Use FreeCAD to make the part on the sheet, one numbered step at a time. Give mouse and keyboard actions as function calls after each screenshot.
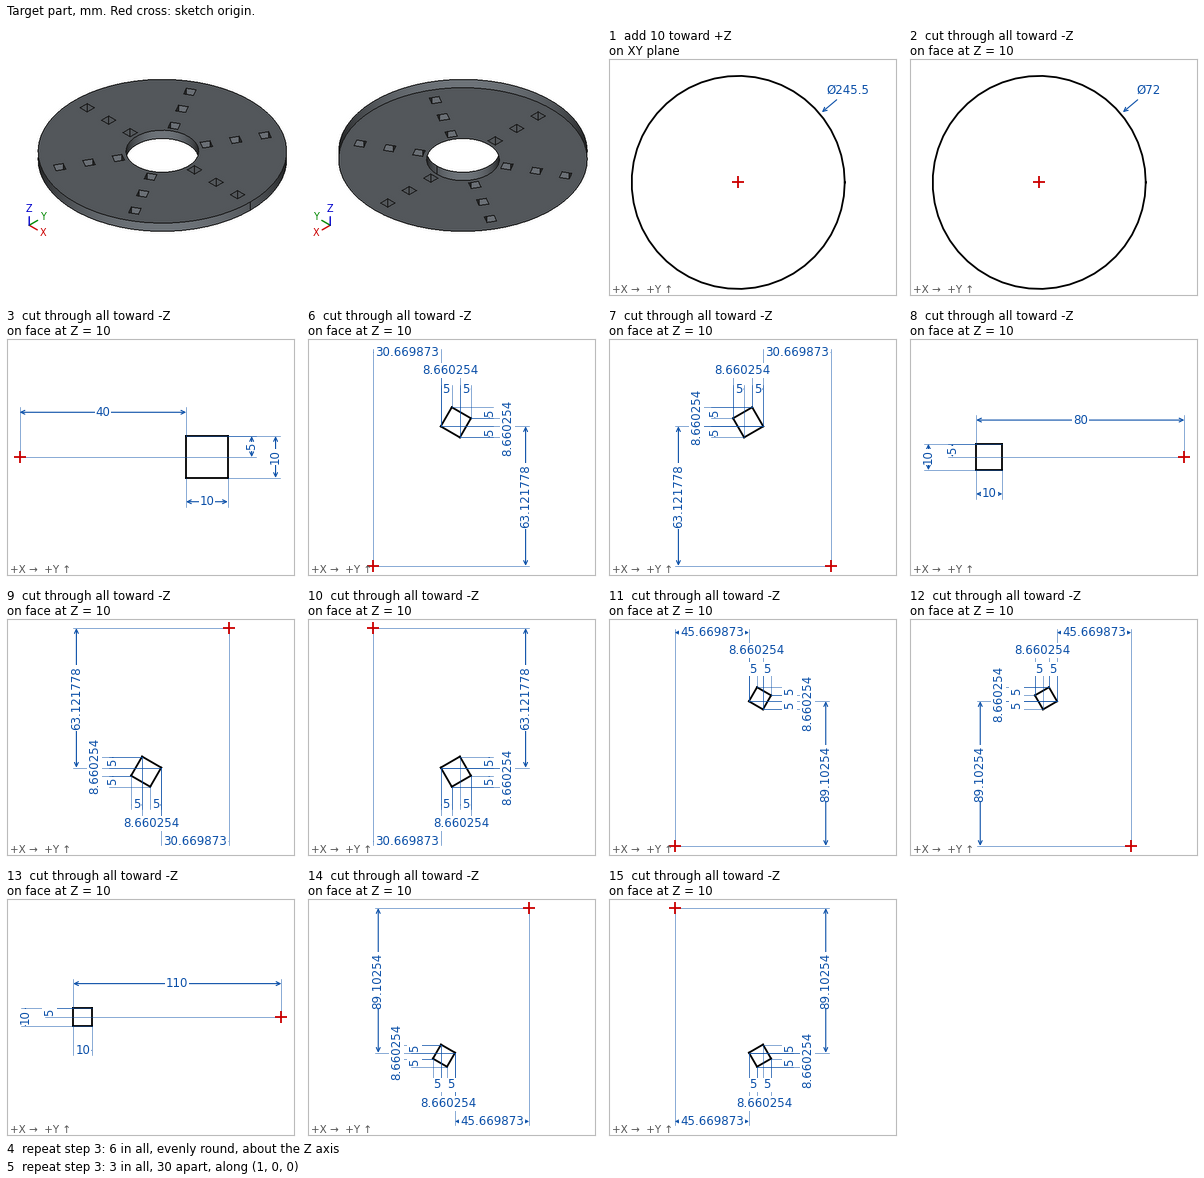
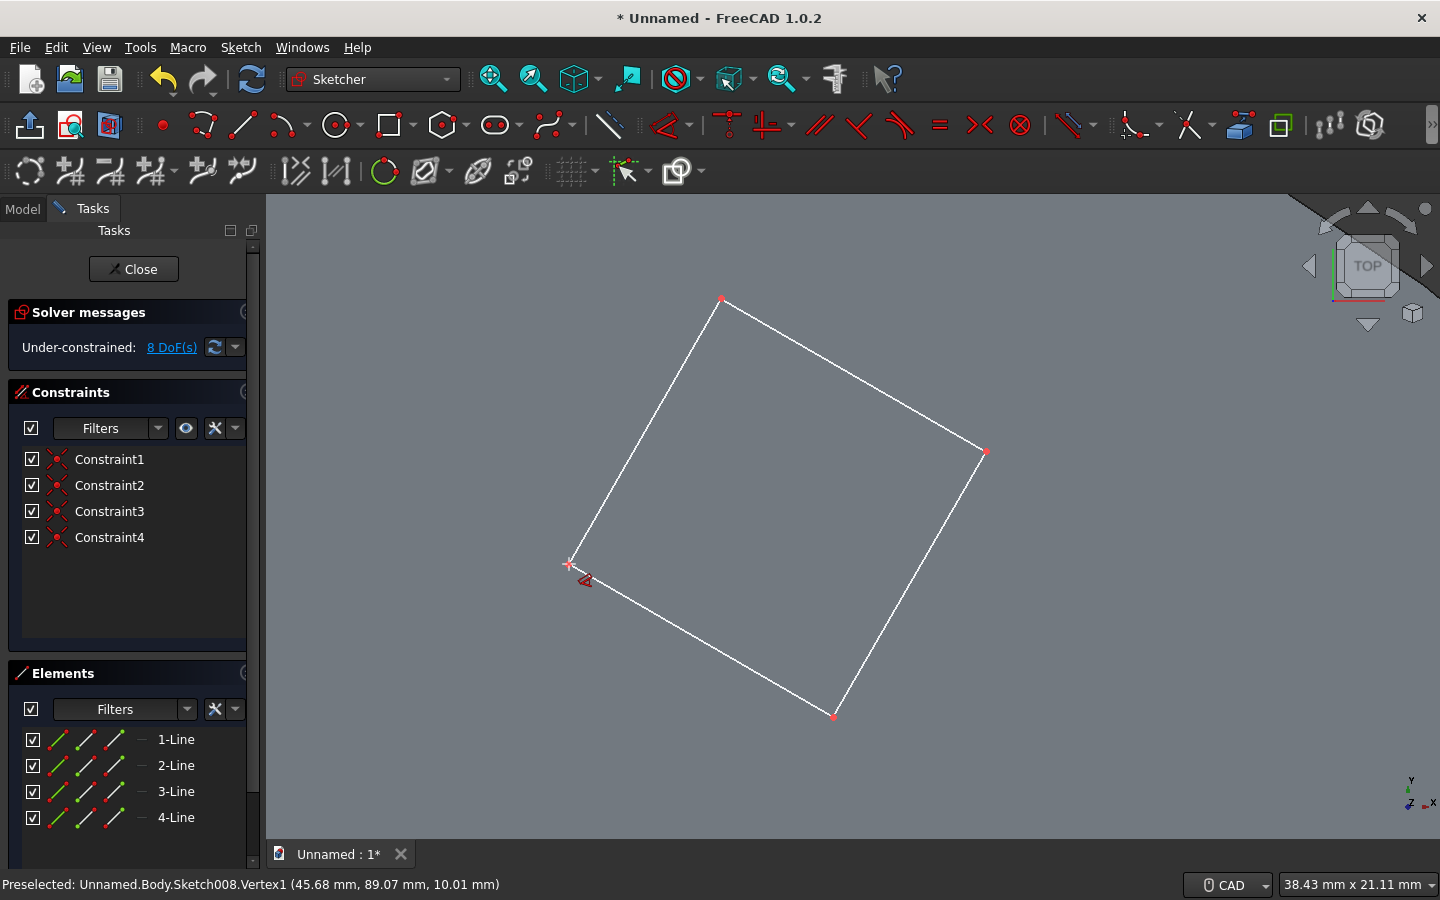
click(648, 610)
click(535, 641)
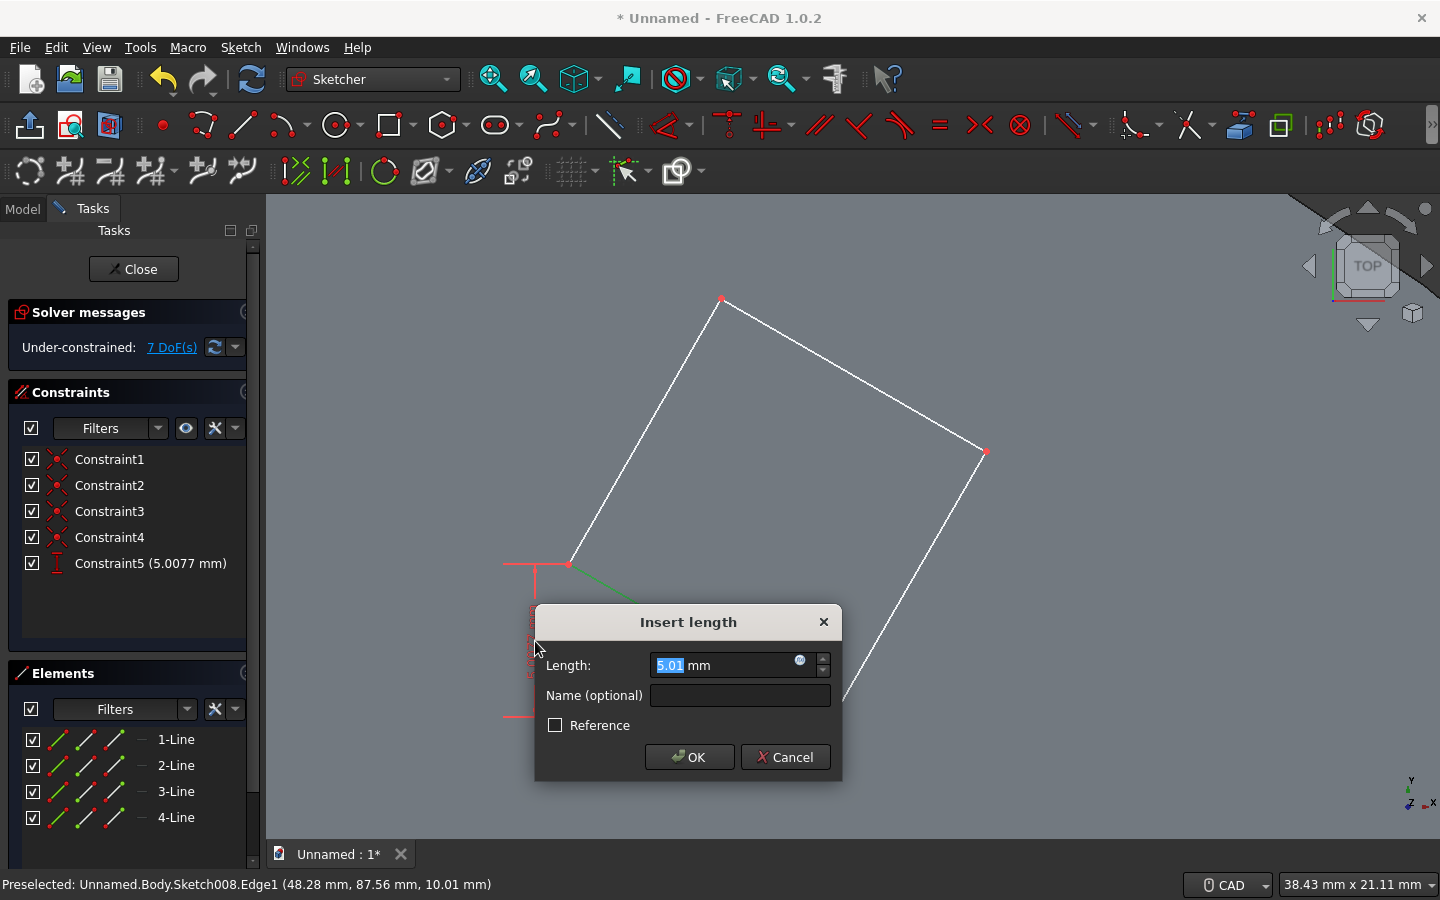
text(5)
key(Return)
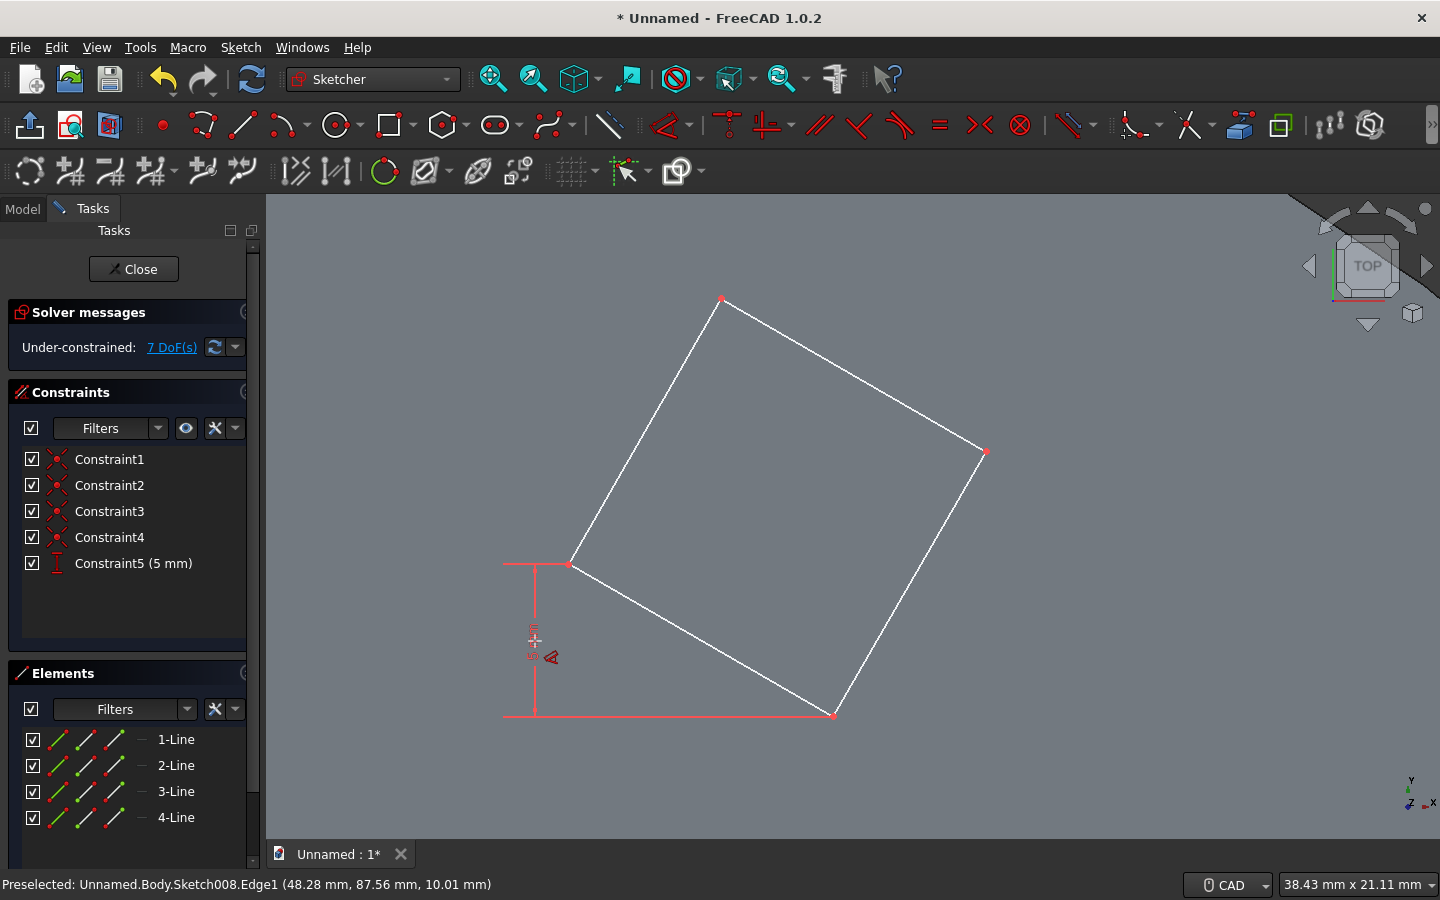
click(879, 637)
click(909, 751)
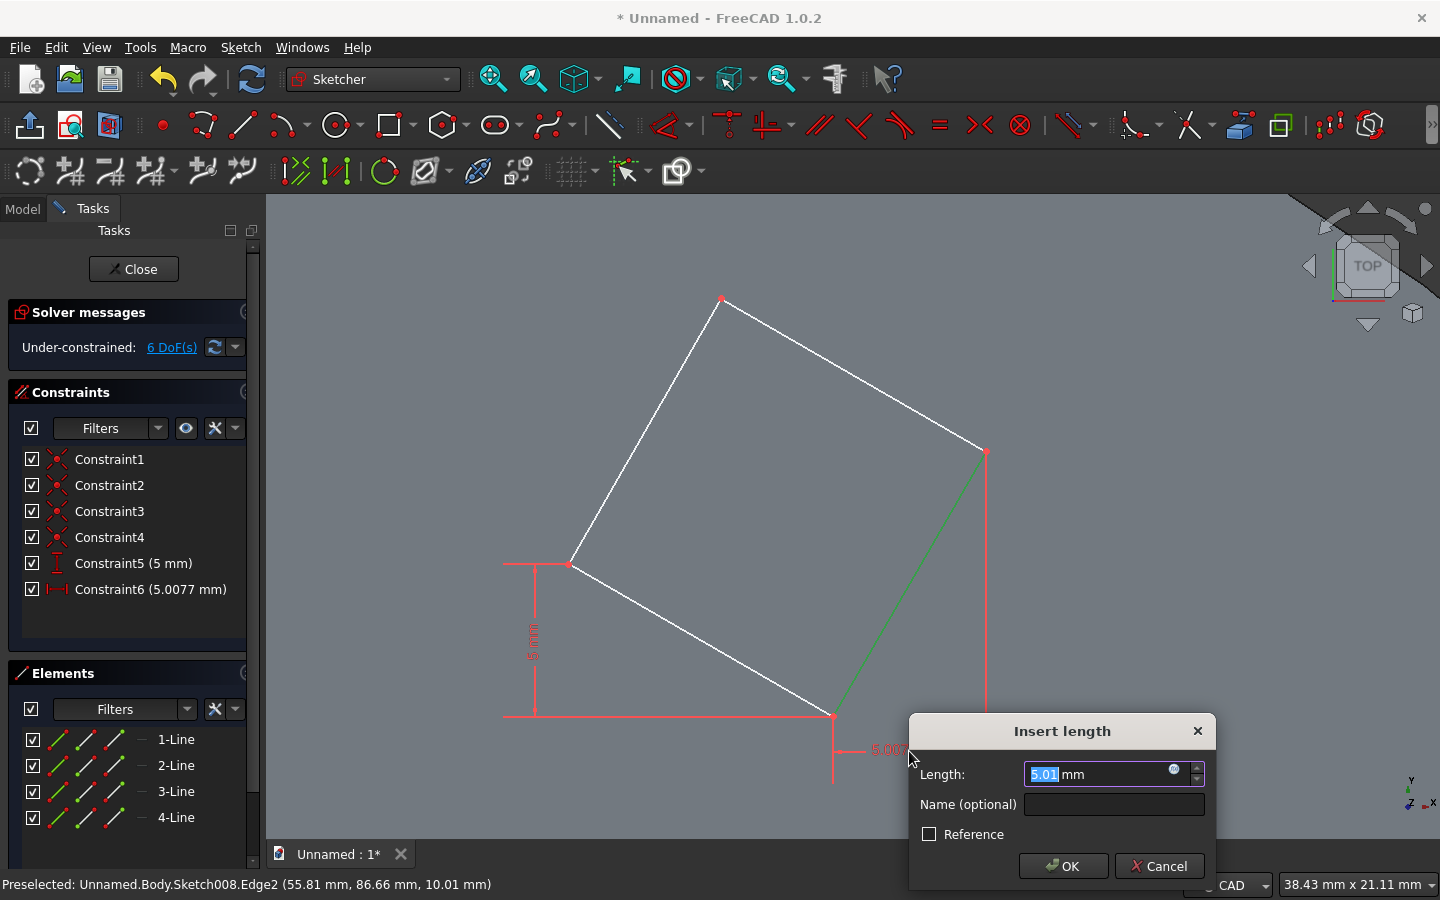
text(5)
key(Return)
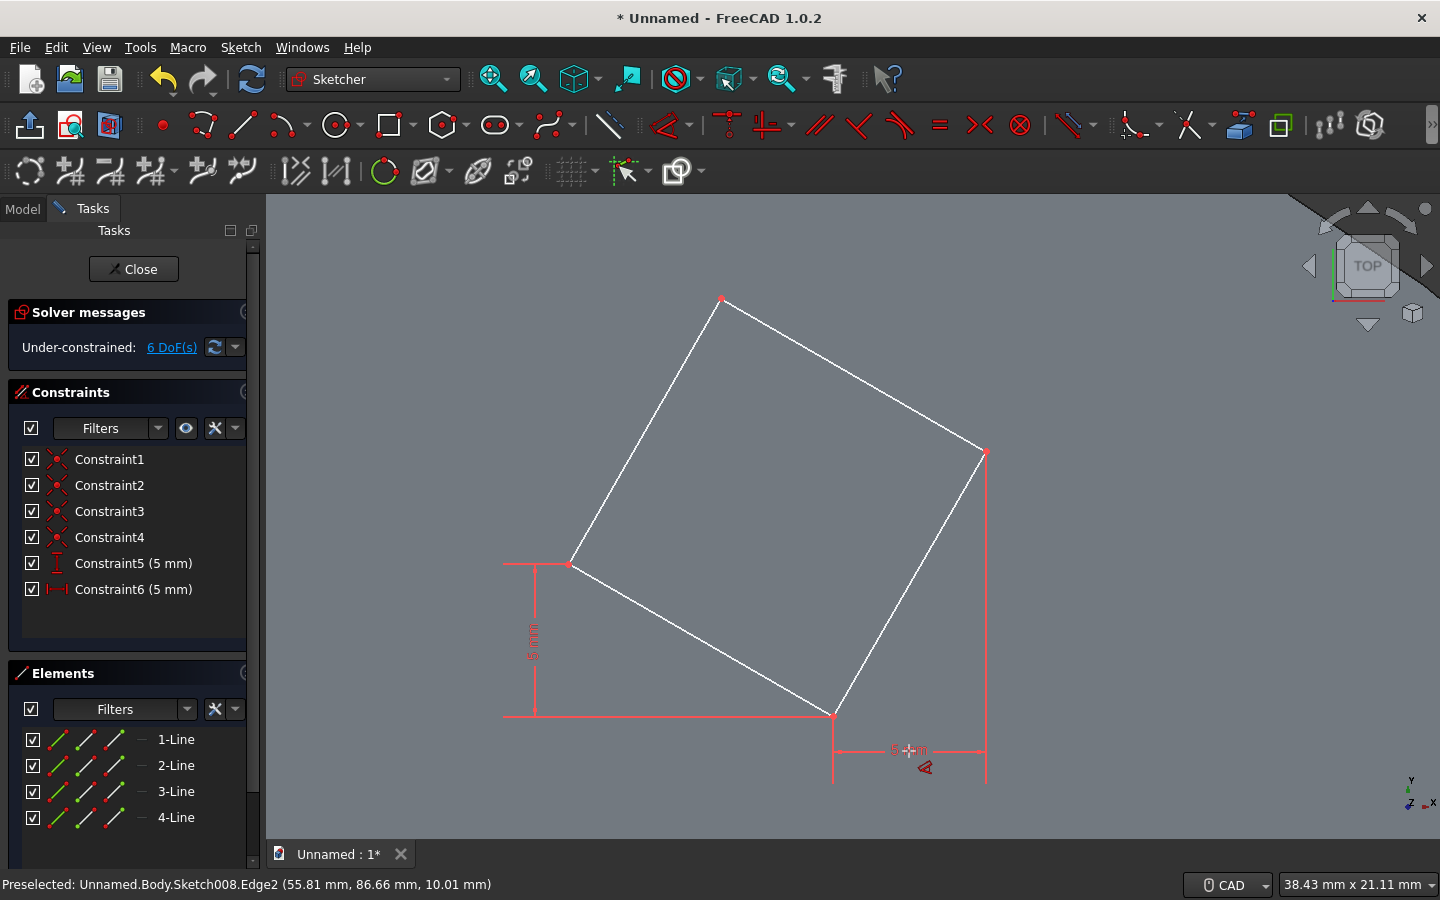
click(907, 406)
click(1020, 375)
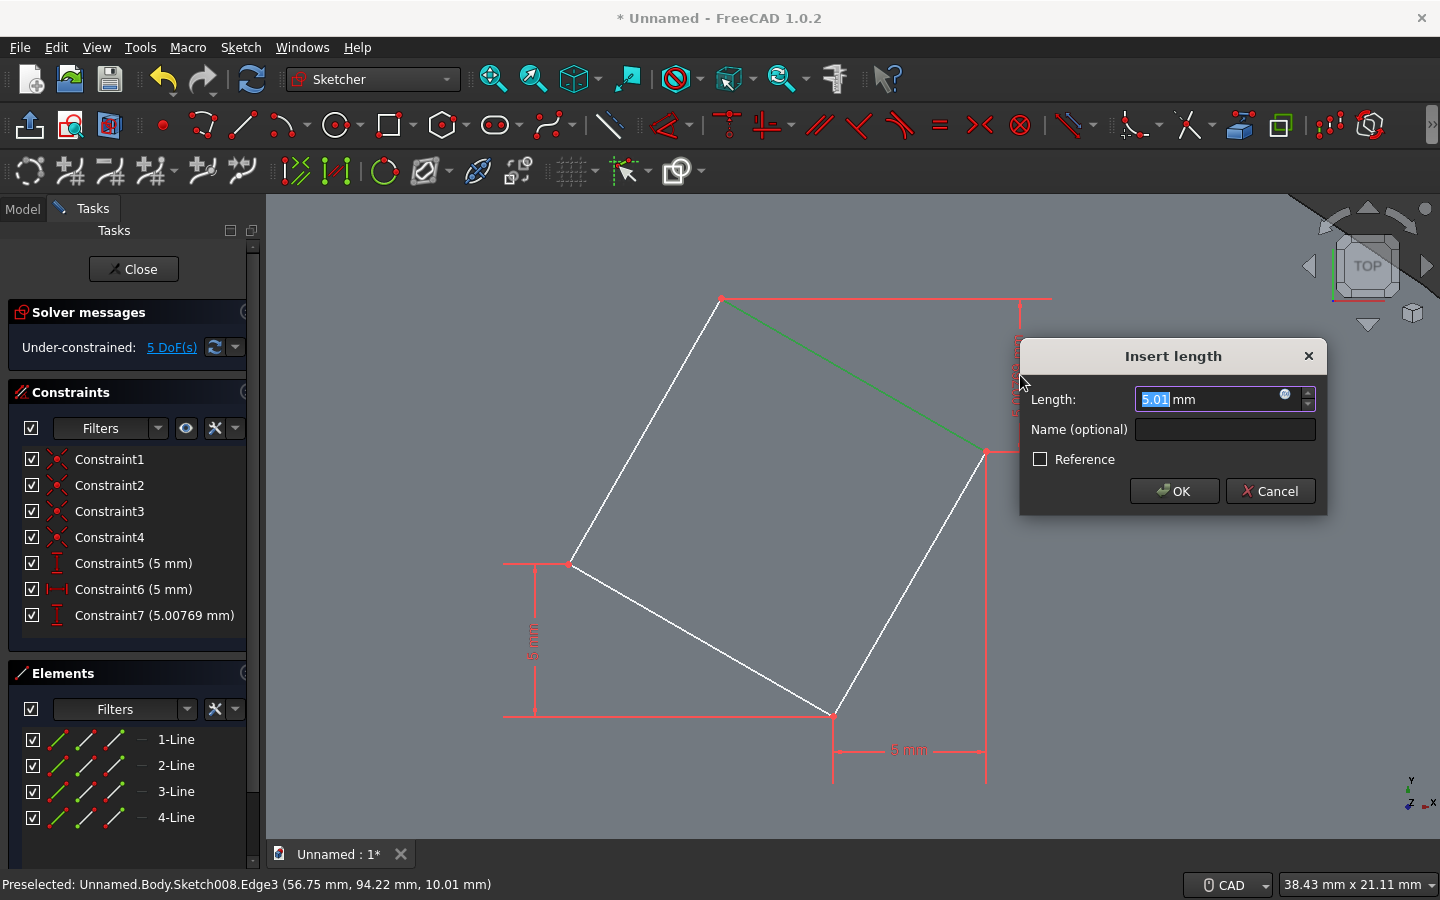
text(5)
key(Return)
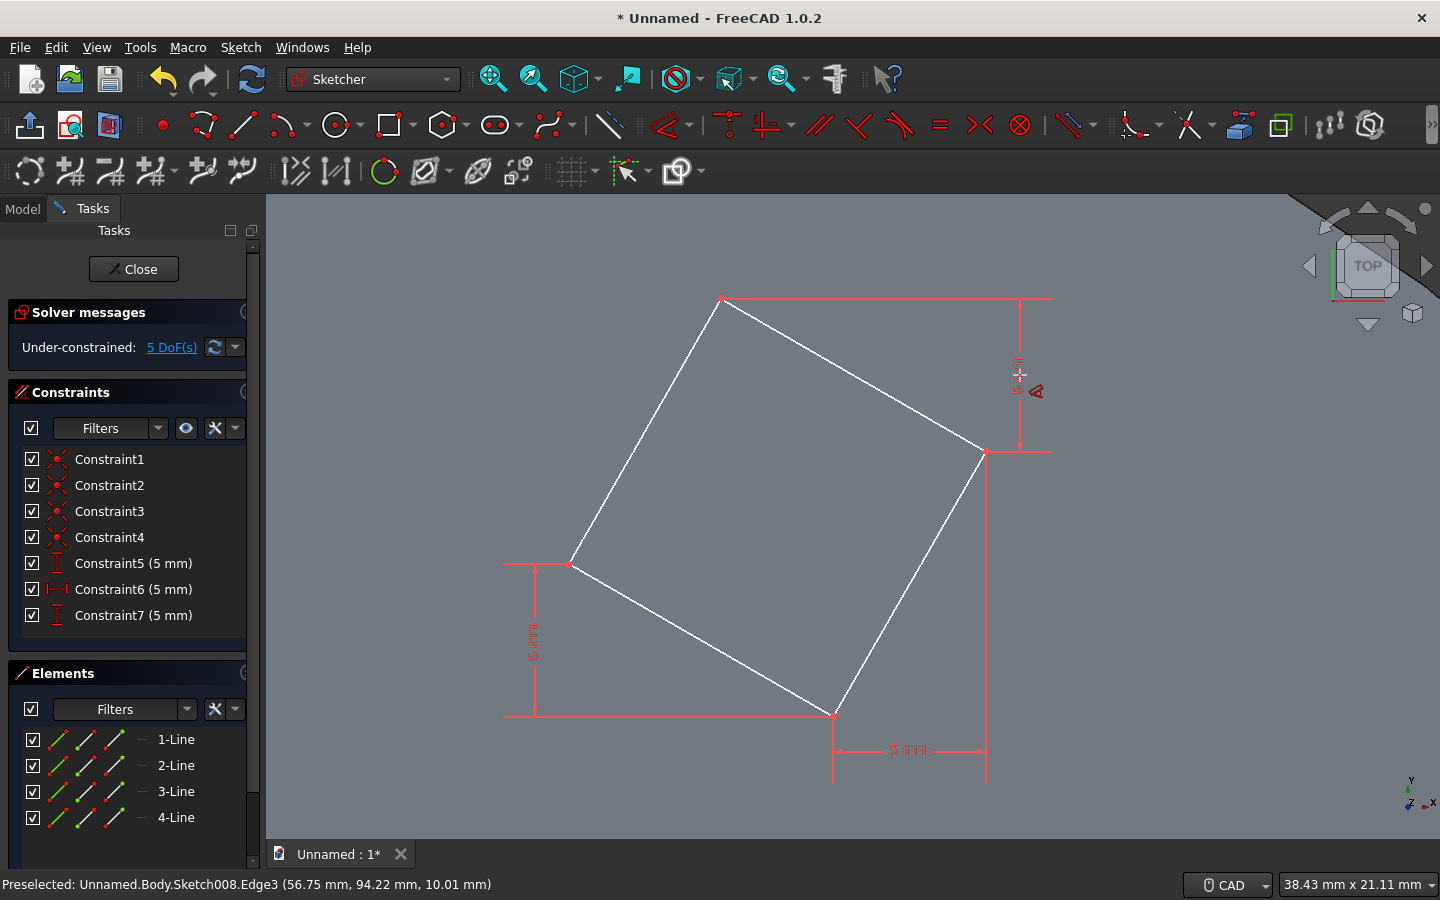
click(675, 379)
click(645, 265)